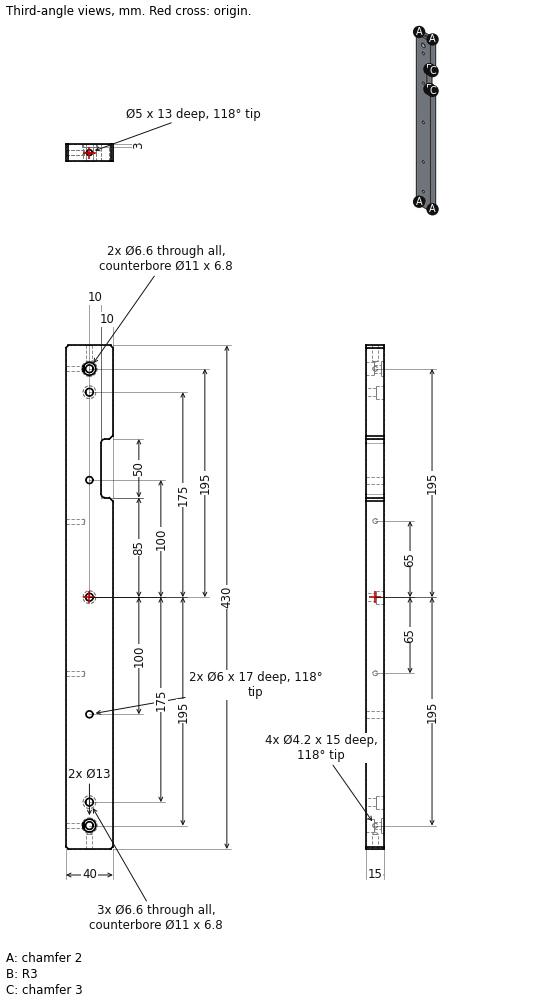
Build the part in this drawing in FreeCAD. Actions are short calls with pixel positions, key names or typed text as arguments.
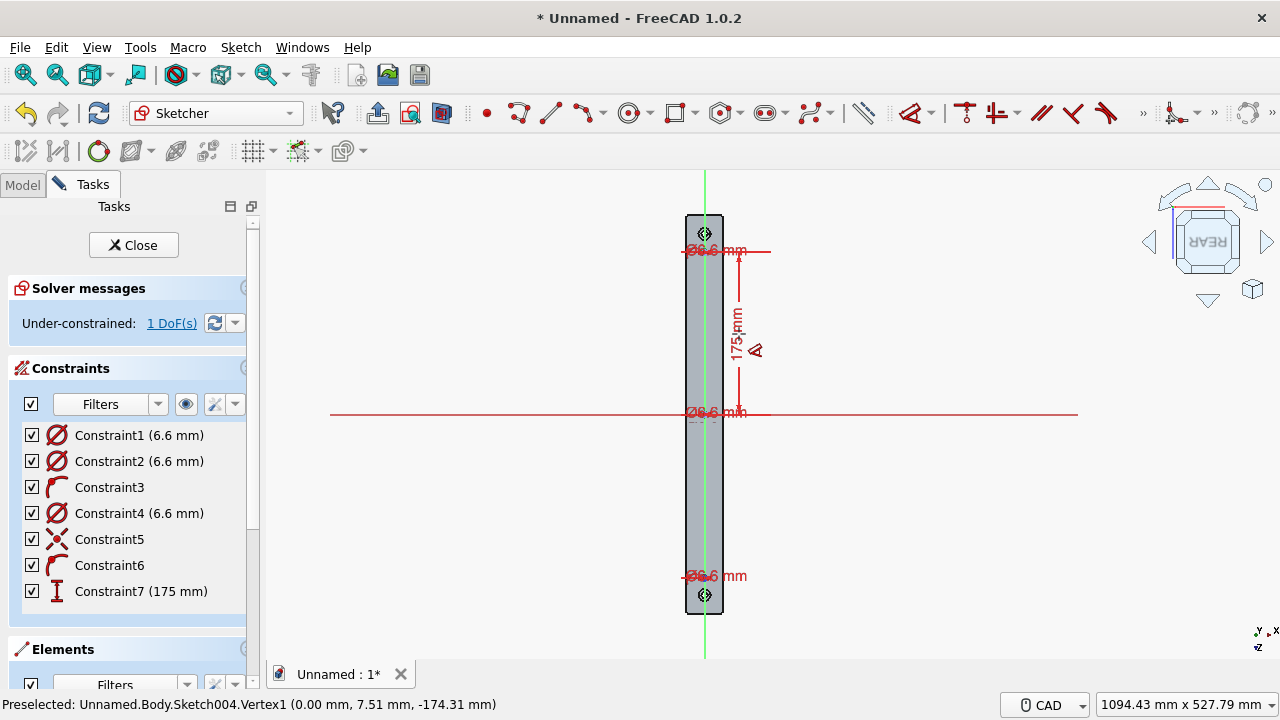
click(705, 578)
click(739, 496)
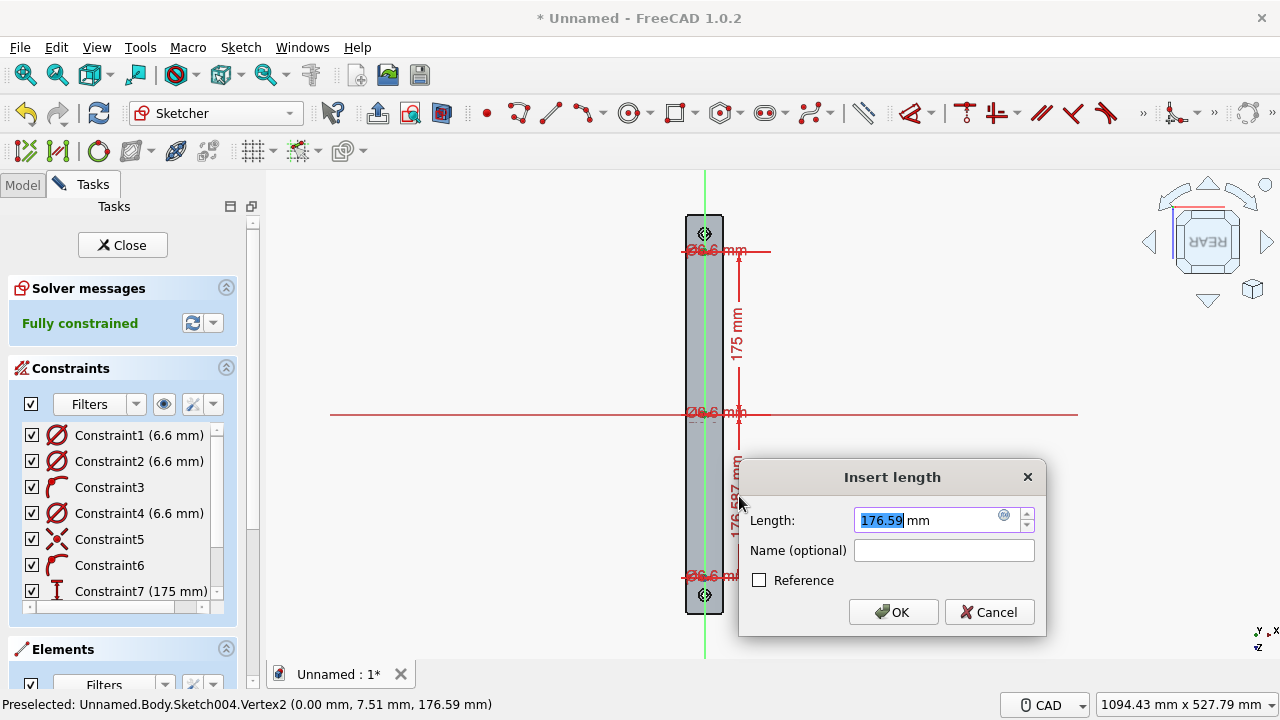
text(175)
key(Return)
key(Escape)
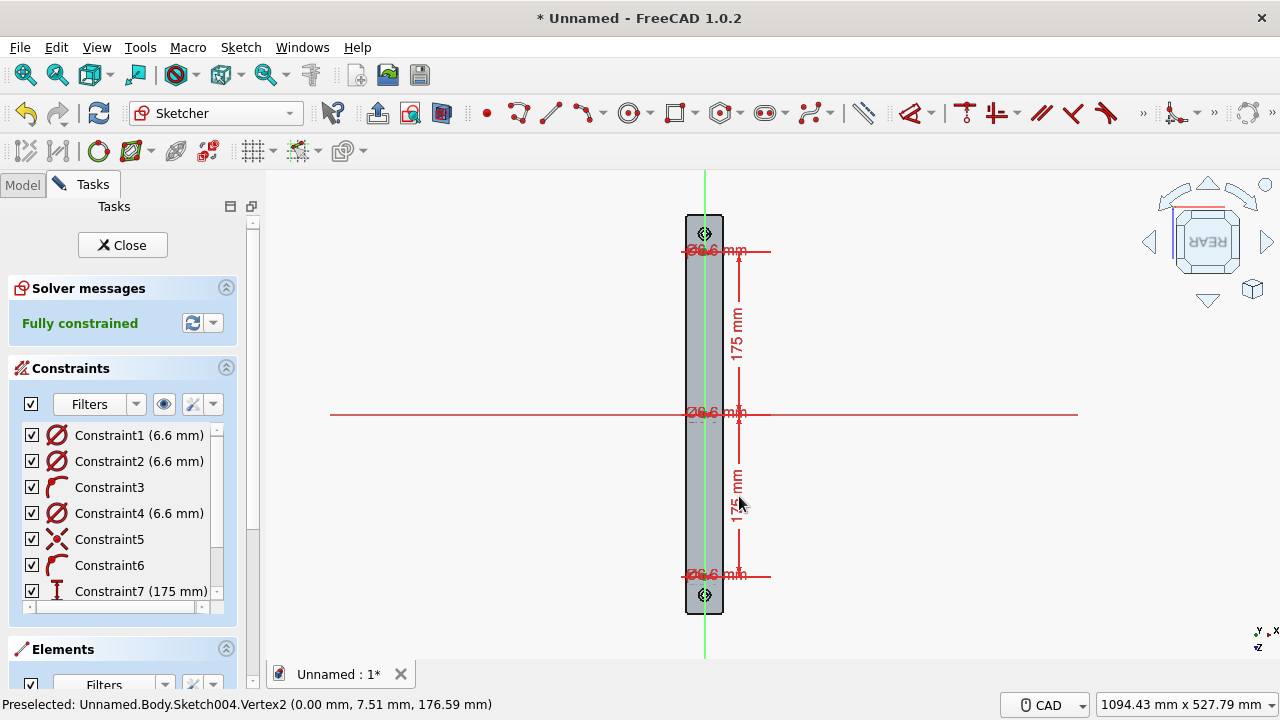
click(123, 245)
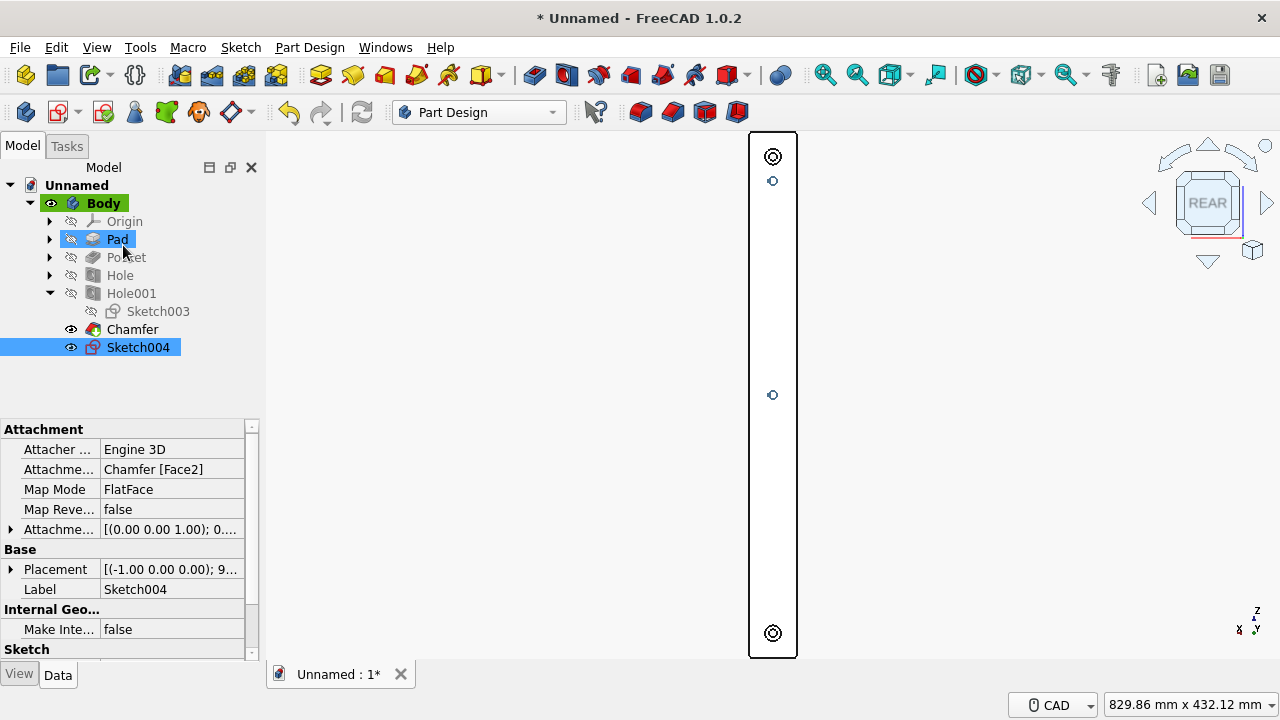
click(568, 76)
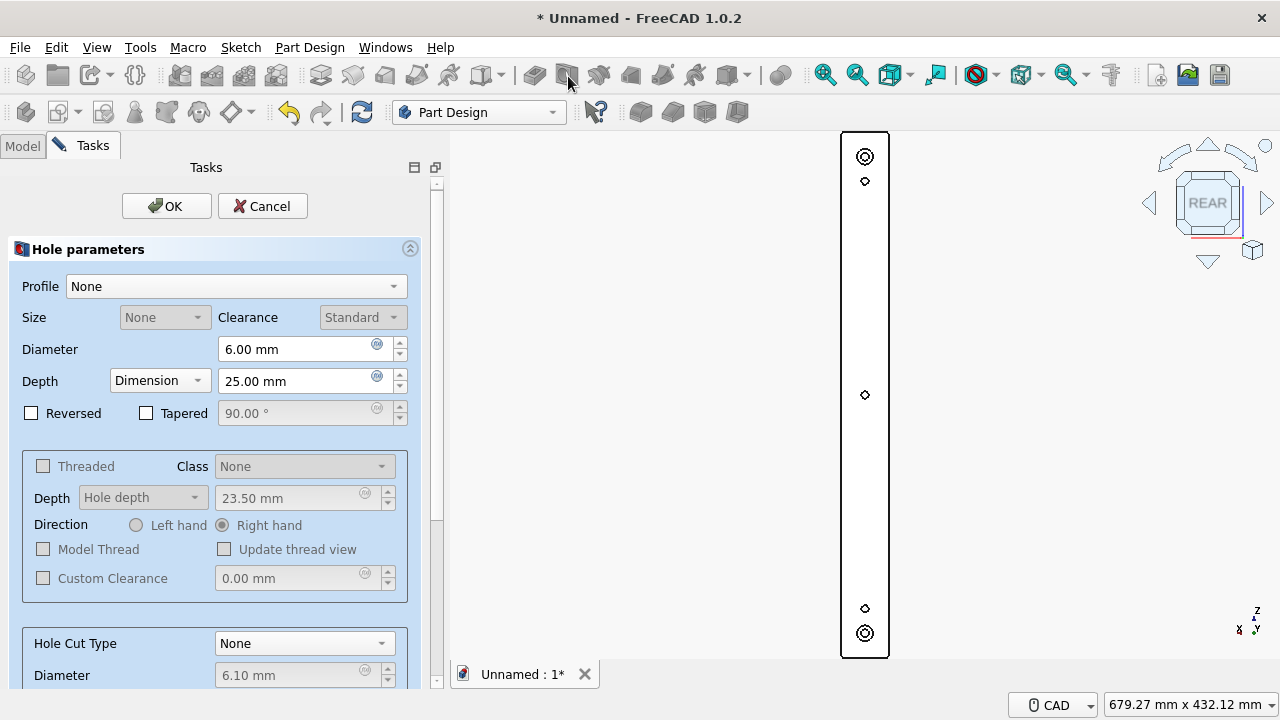
triple_click(305, 349)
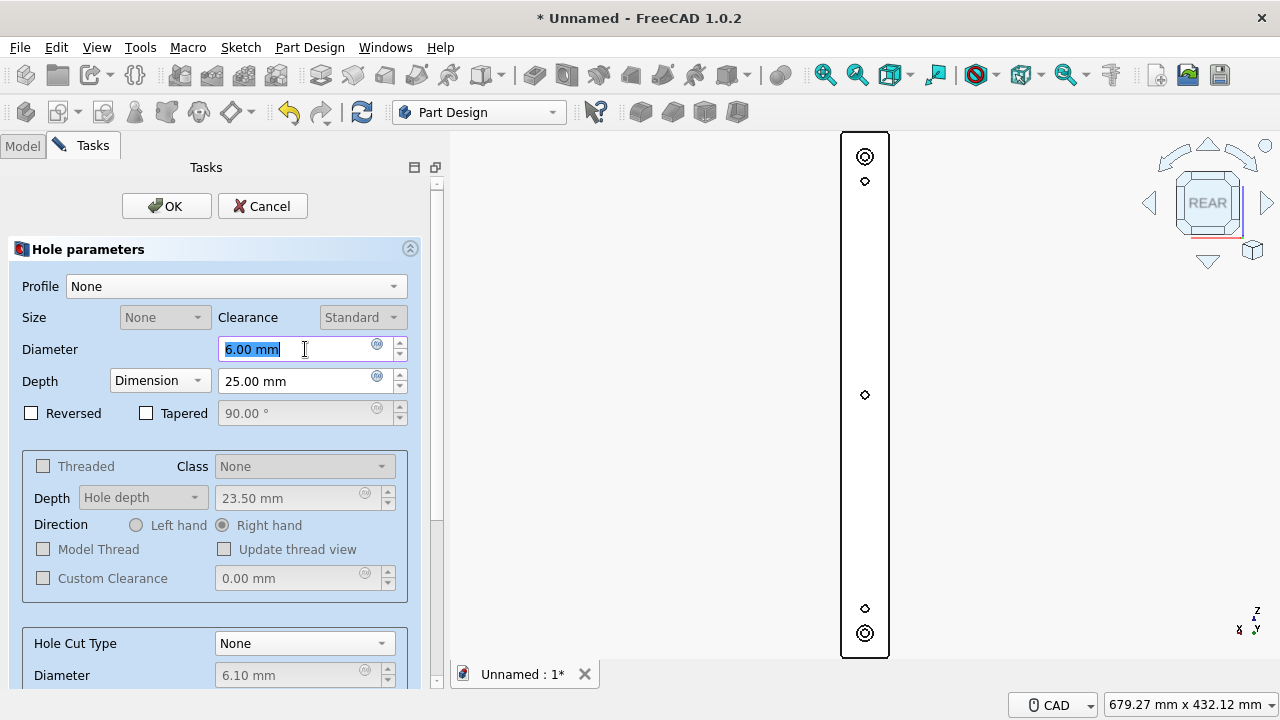
text(6.6)
key(Tab)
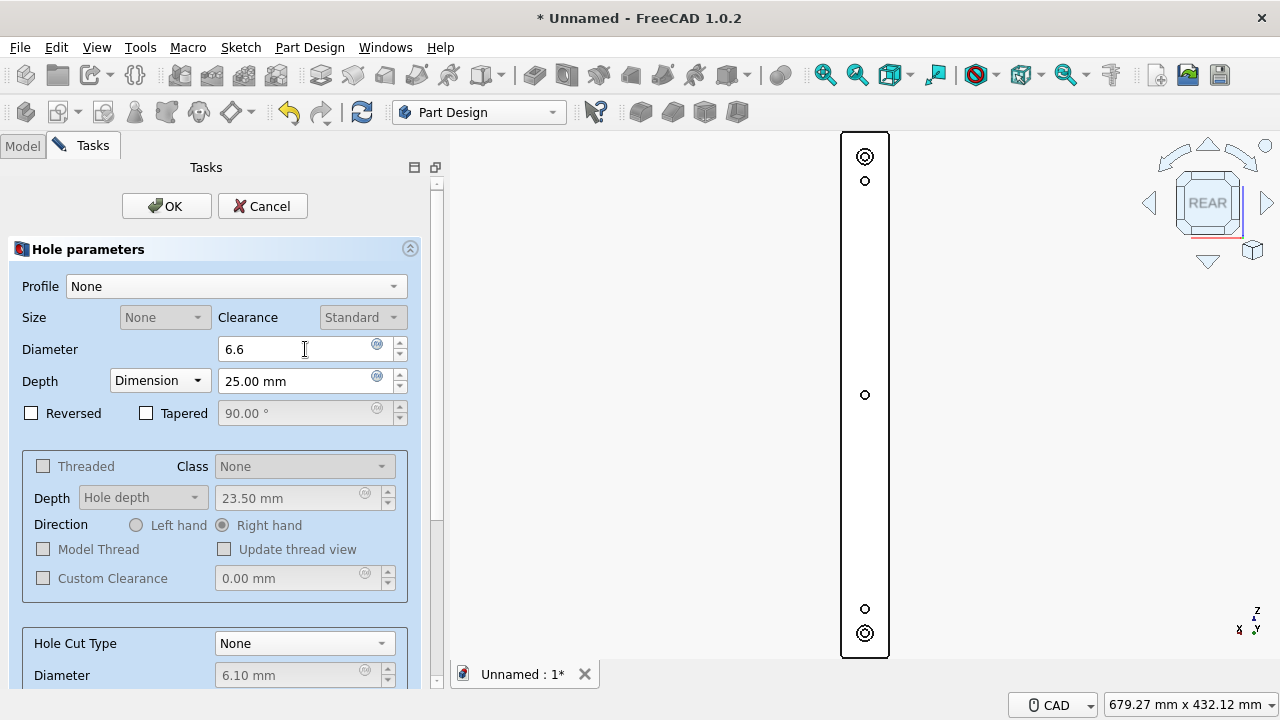
click(161, 380)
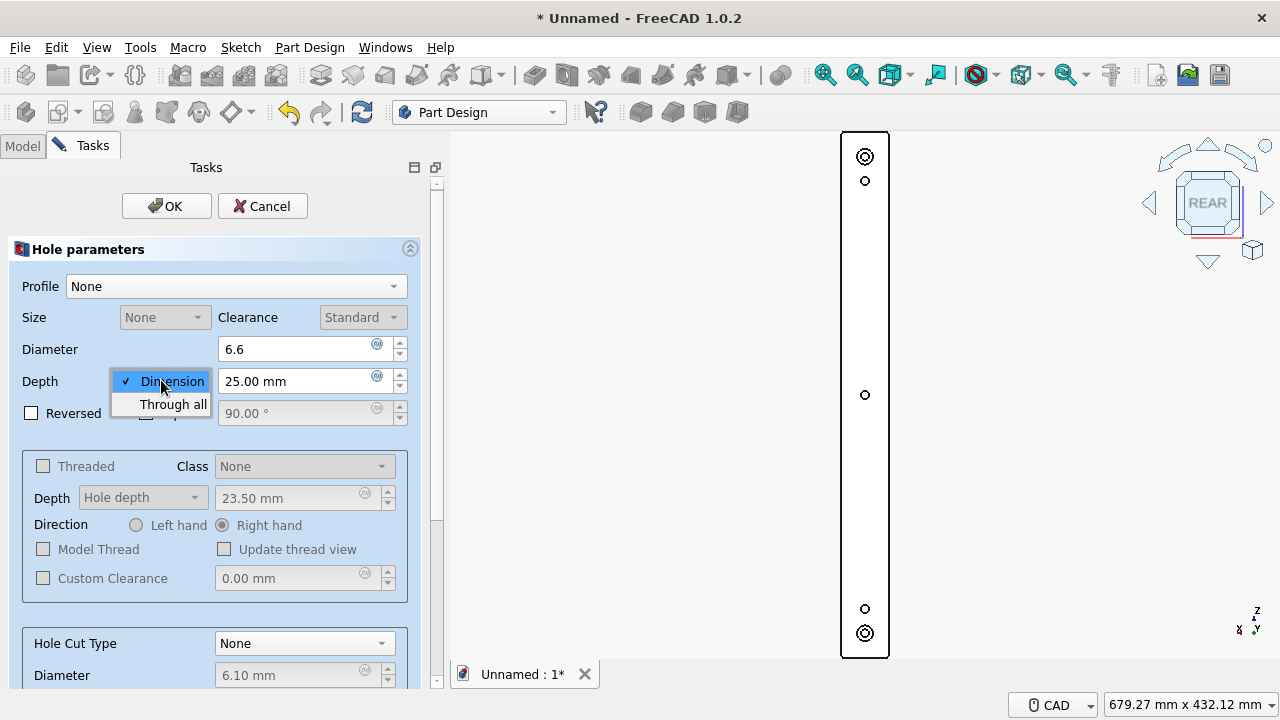
click(160, 404)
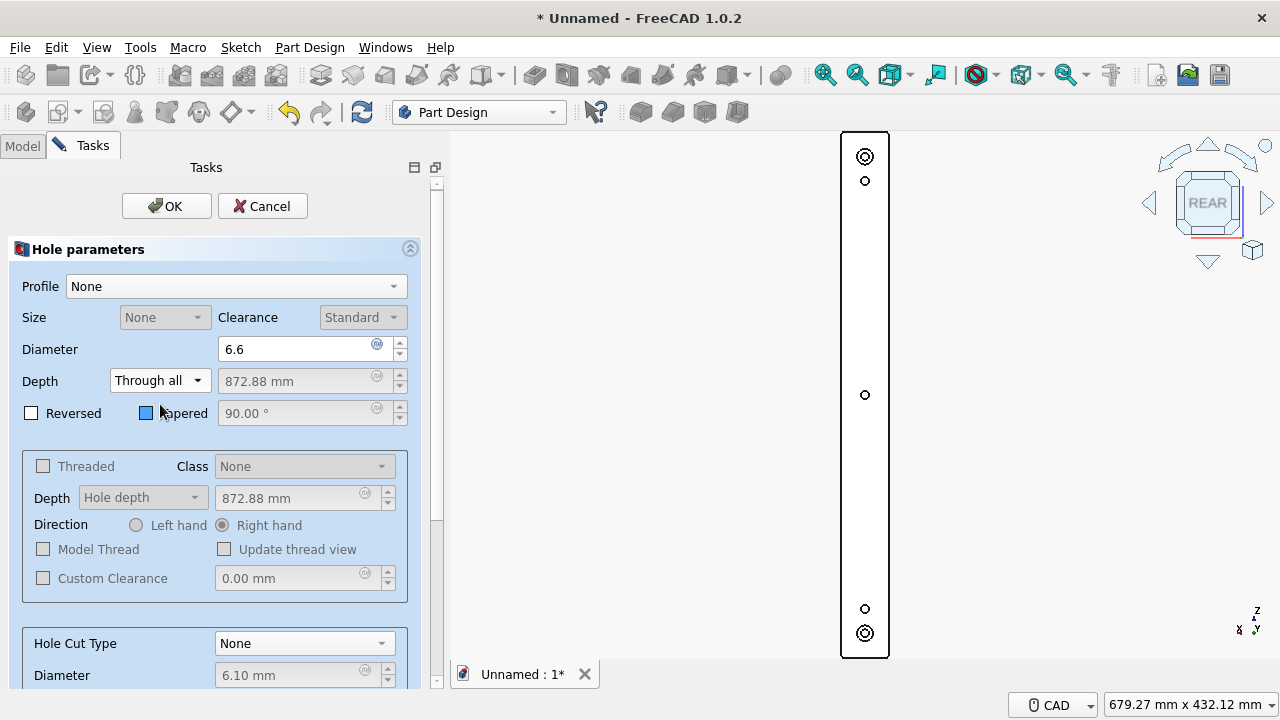
click(306, 644)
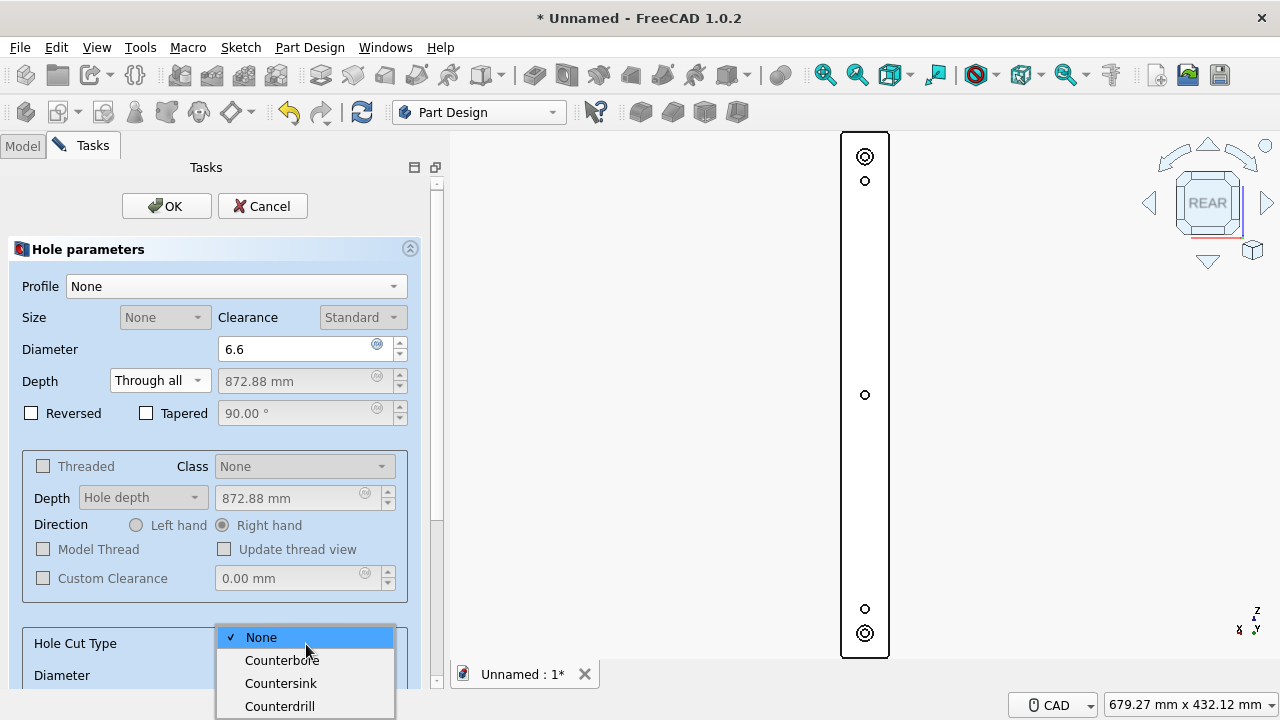
click(304, 660)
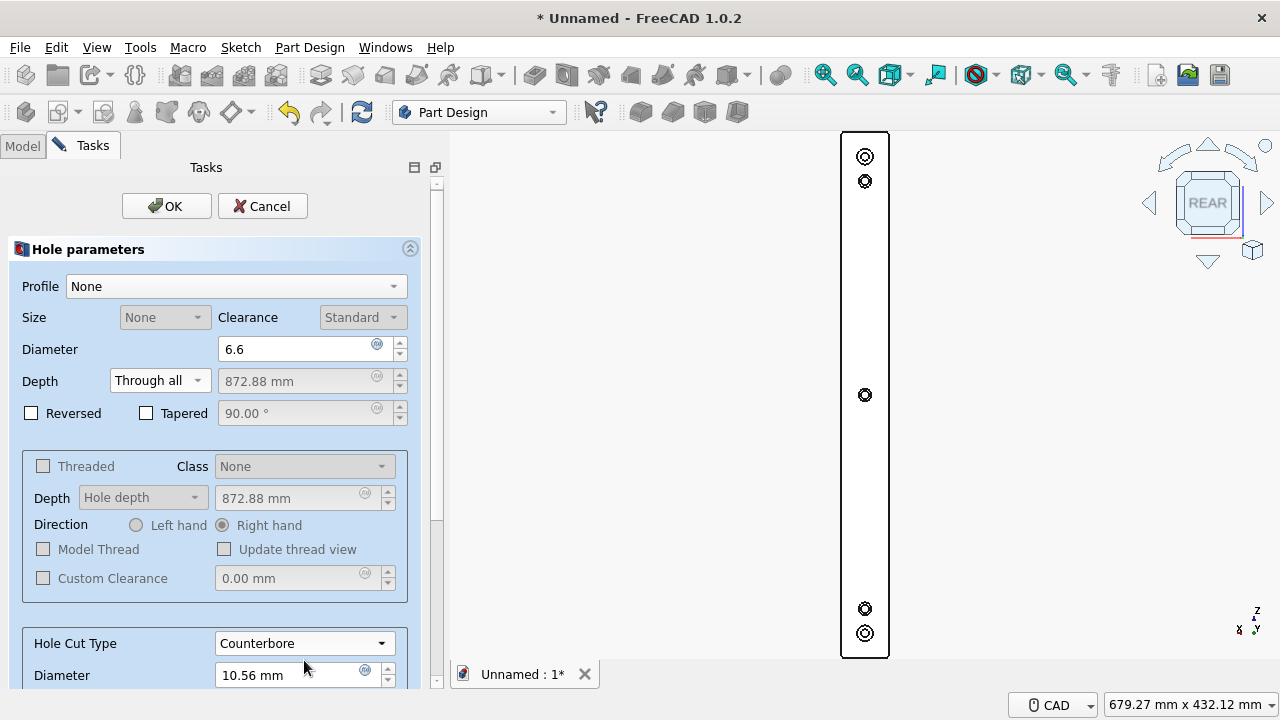
triple_click(298, 675)